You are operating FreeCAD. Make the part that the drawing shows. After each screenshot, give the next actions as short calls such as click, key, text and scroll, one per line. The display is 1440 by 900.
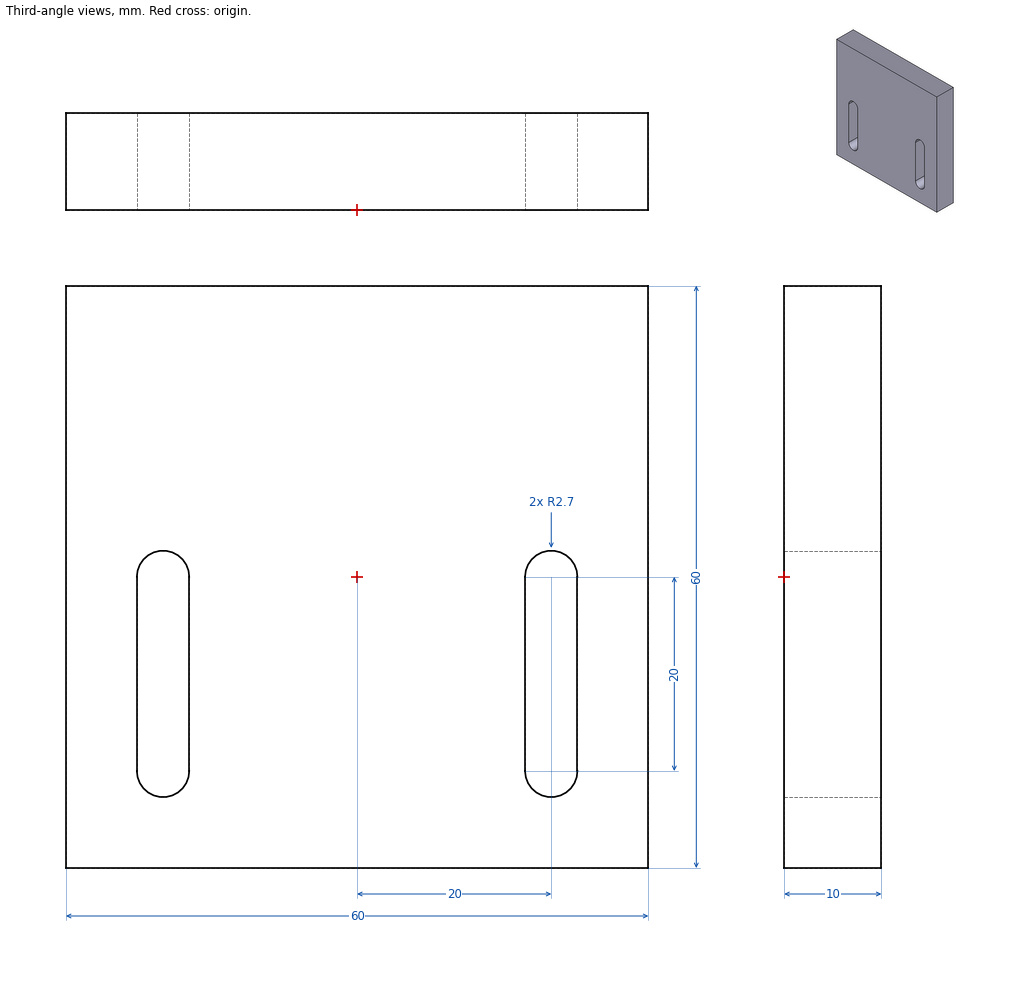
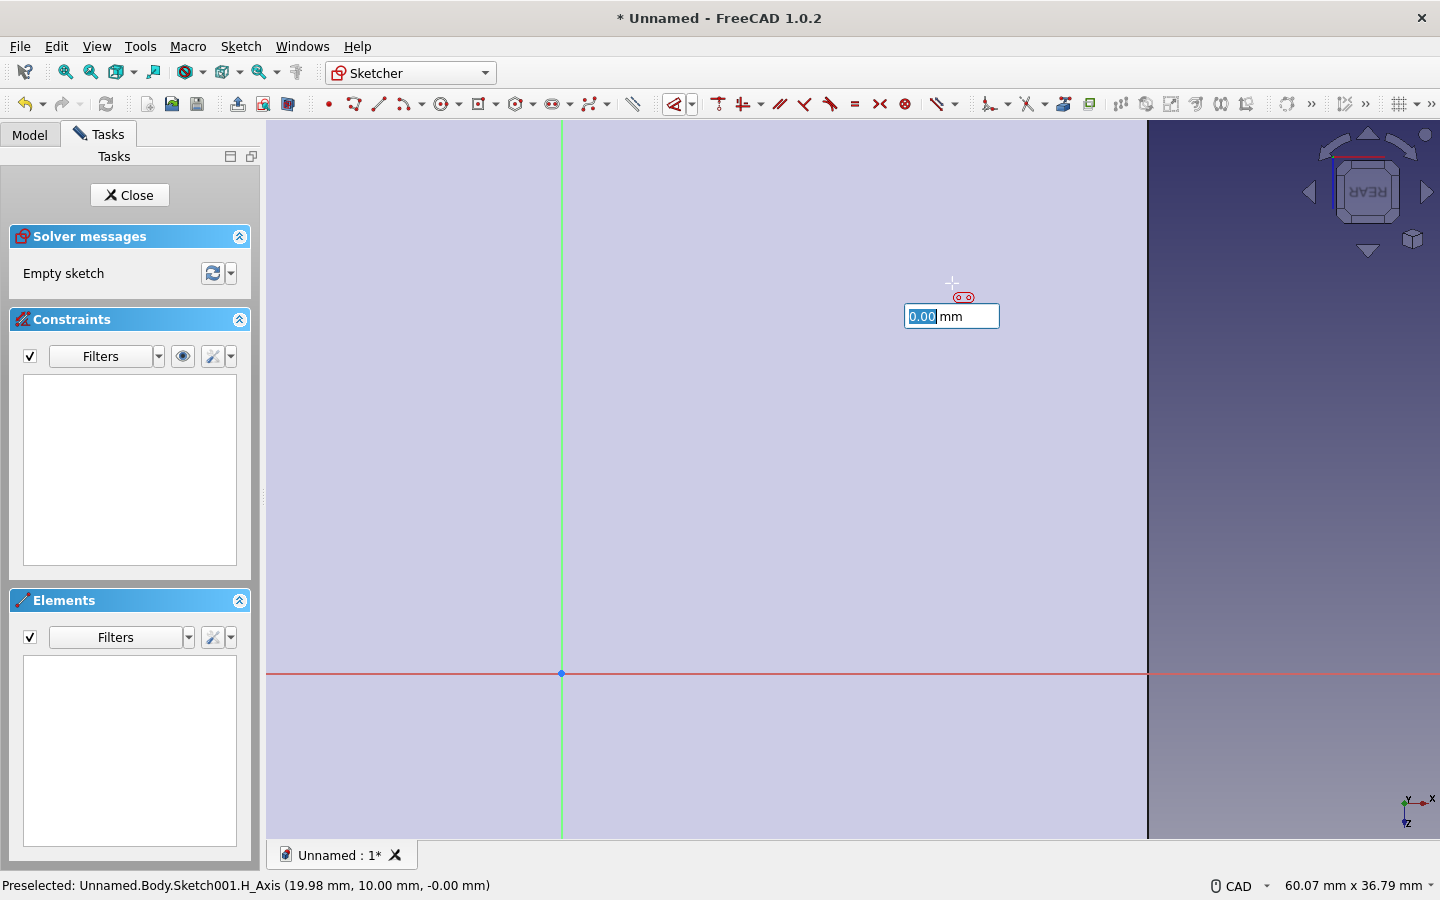
click(900, 478)
key(Escape)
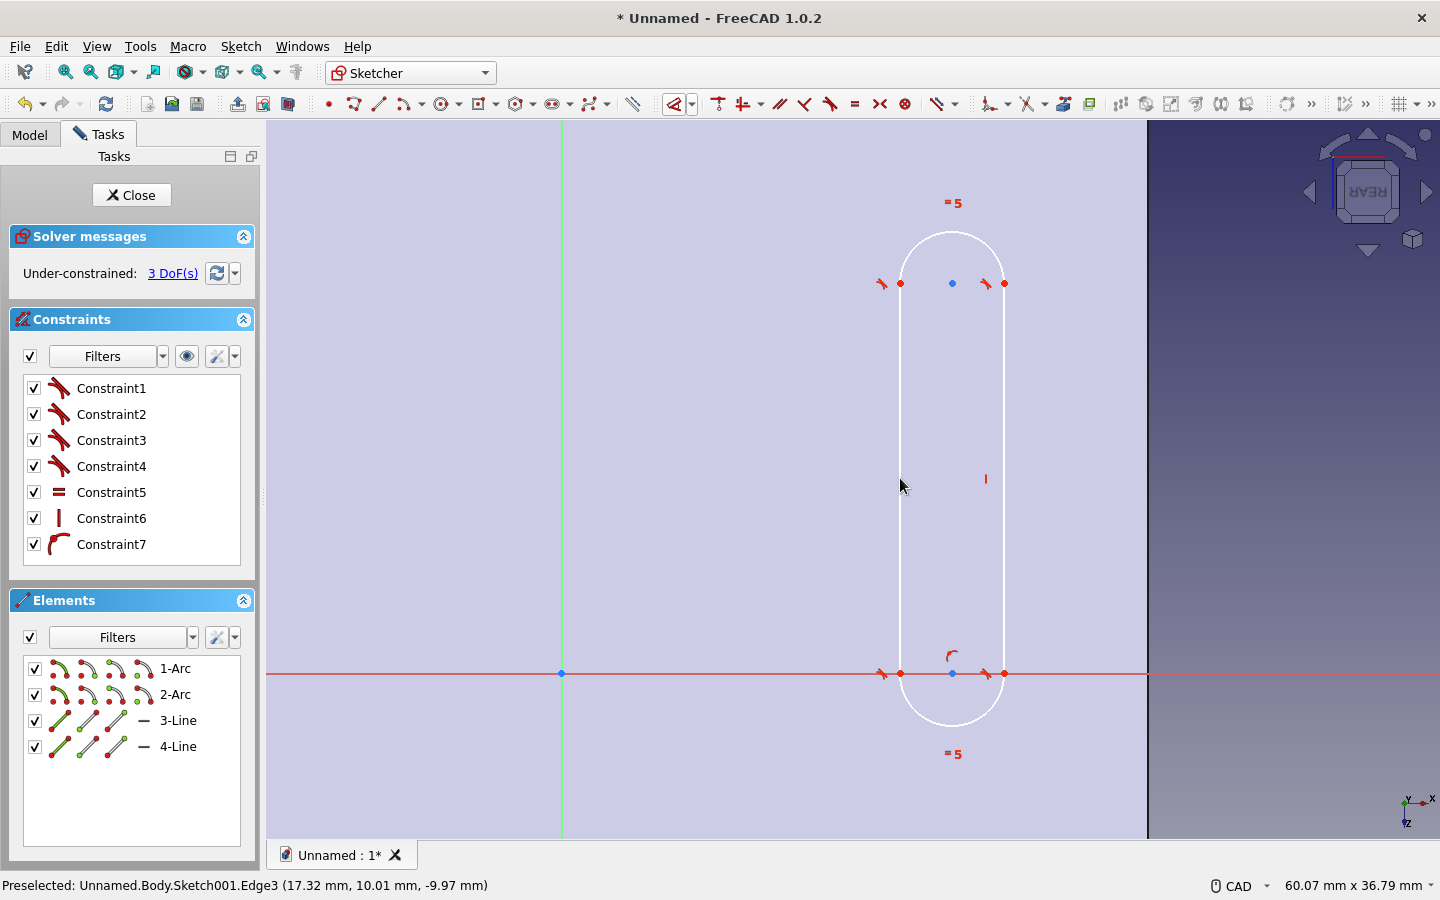
click(921, 716)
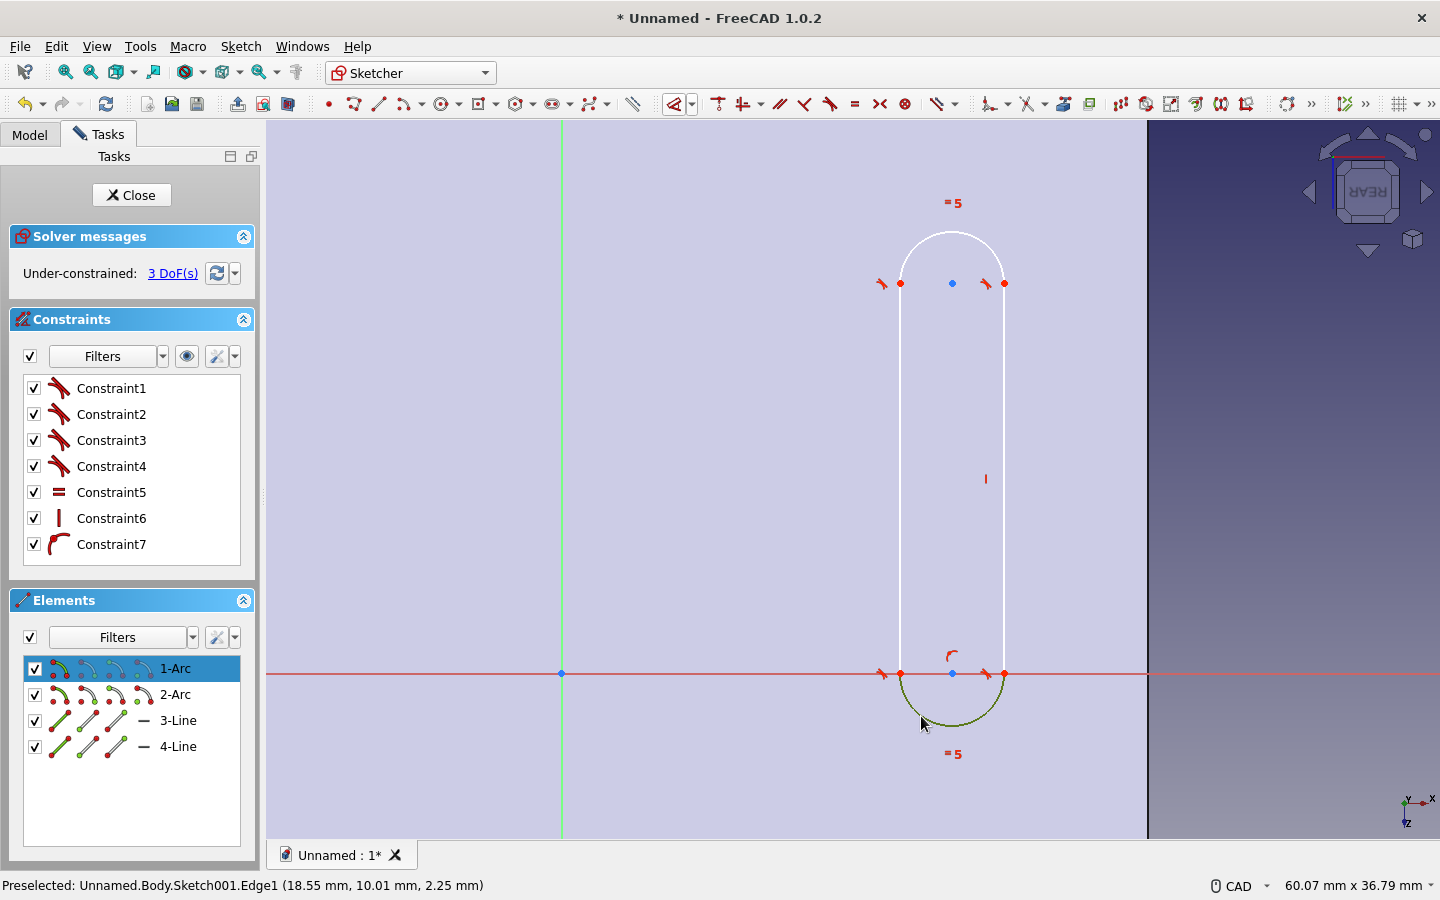
key(k)
key(r)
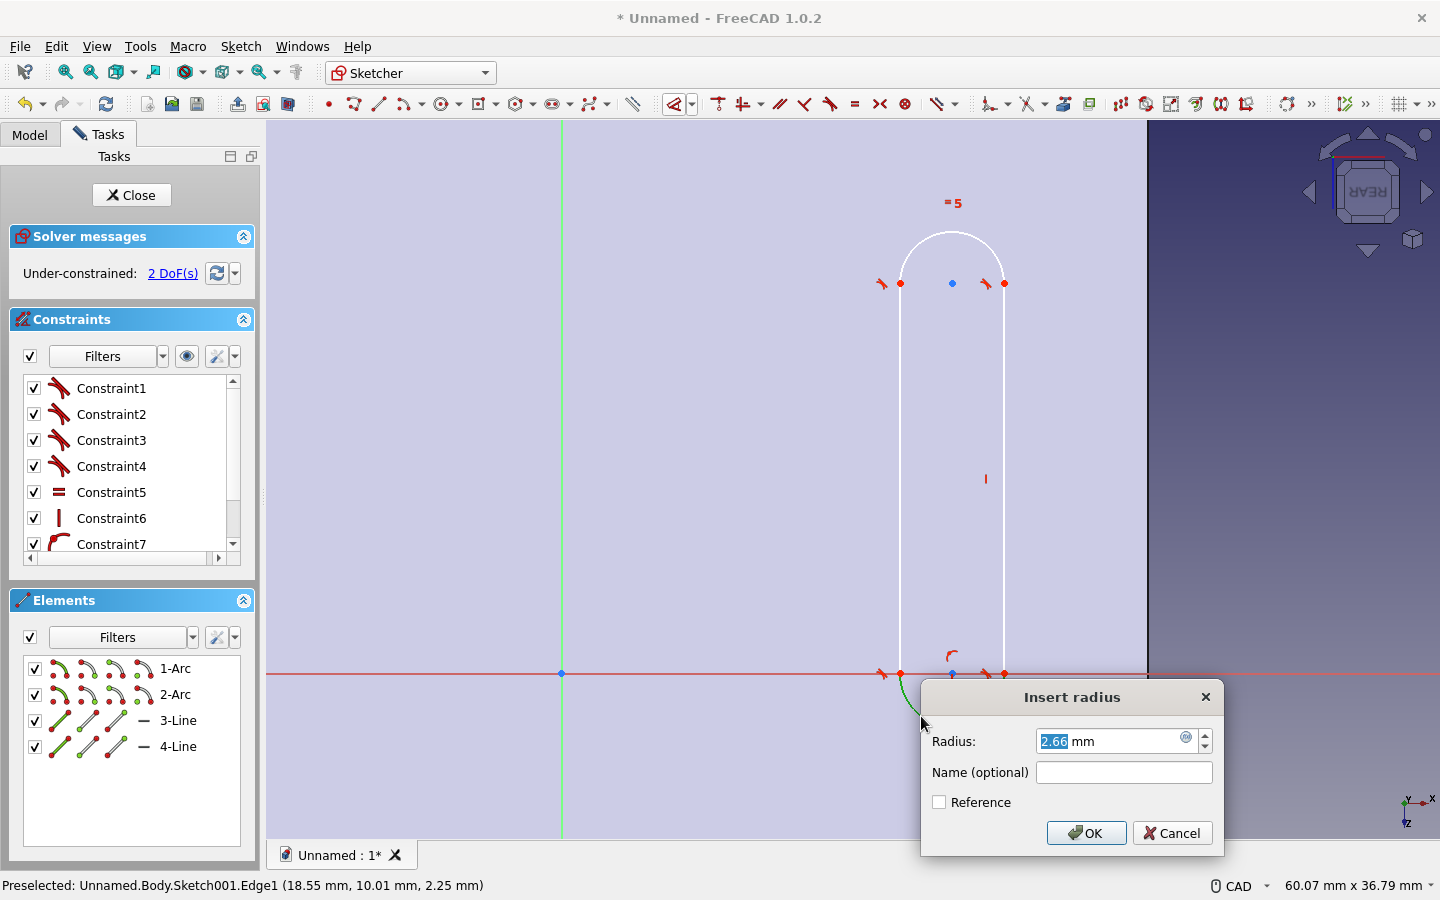
text(2.7)
key(Return)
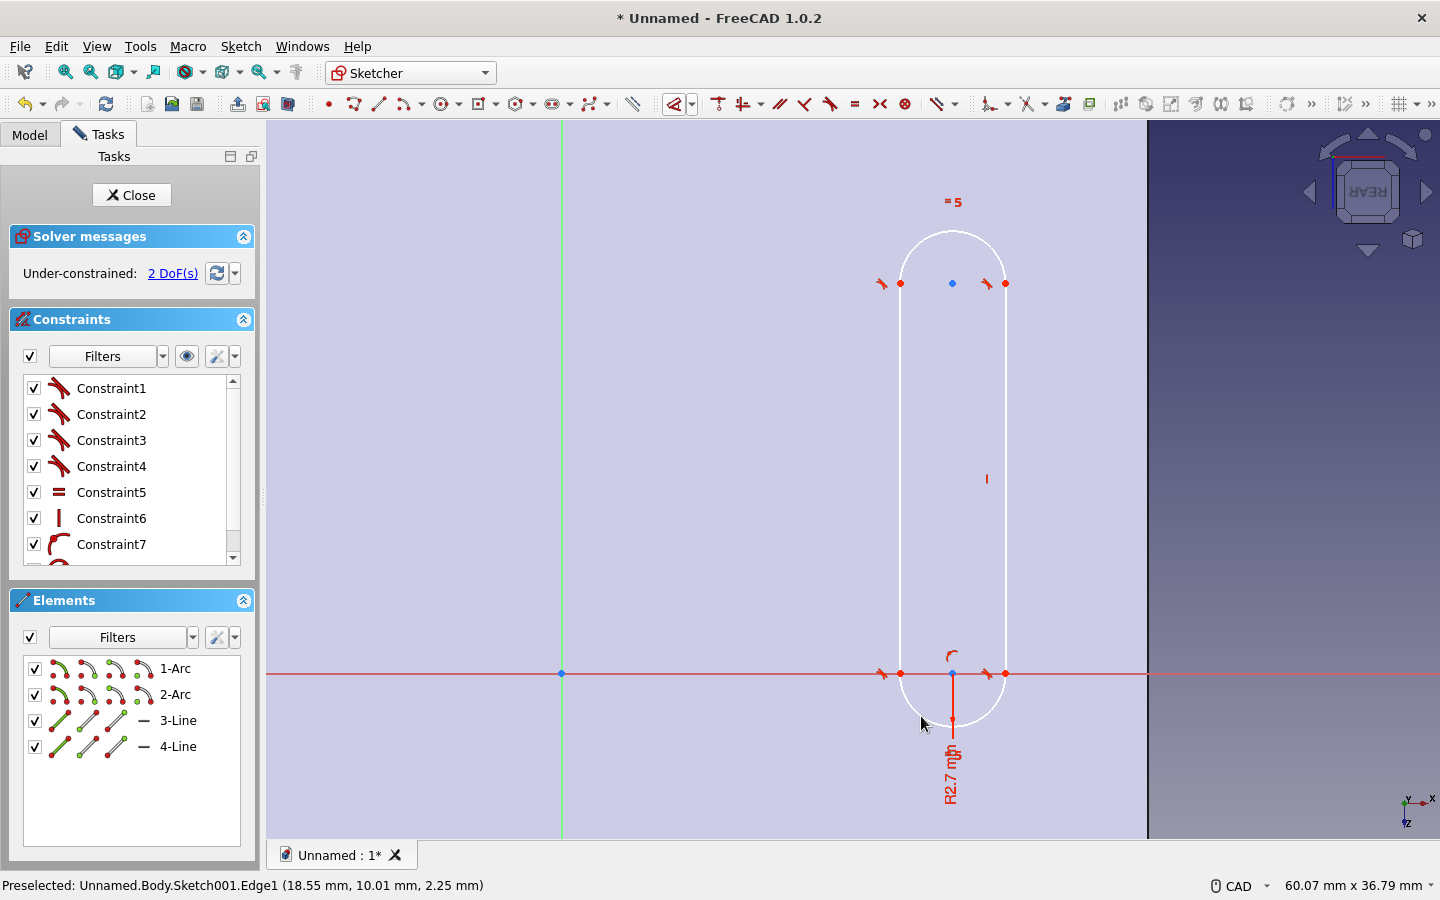
click(900, 557)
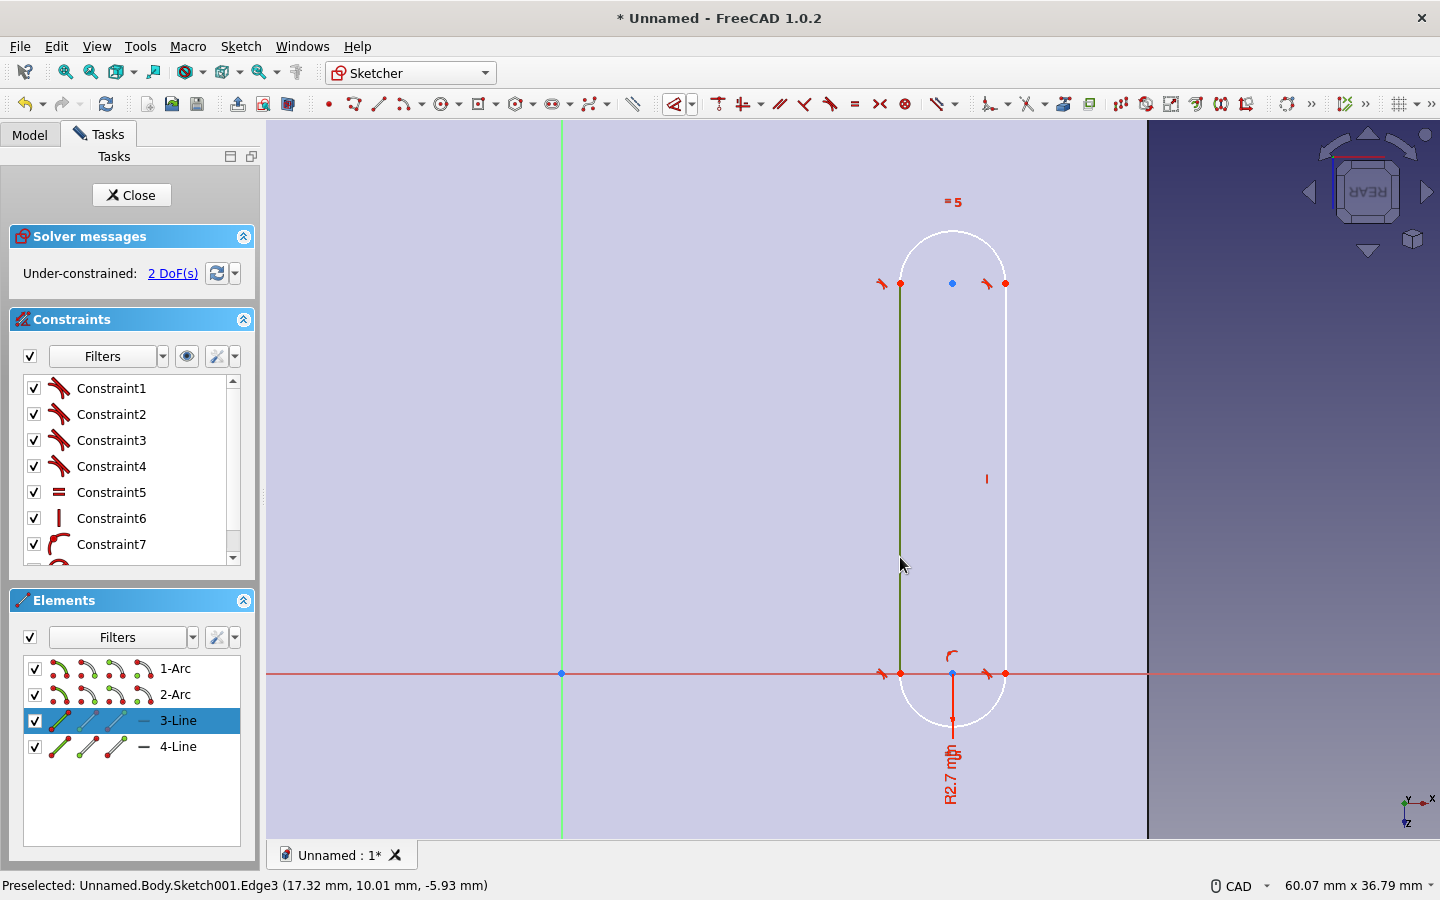
key(i)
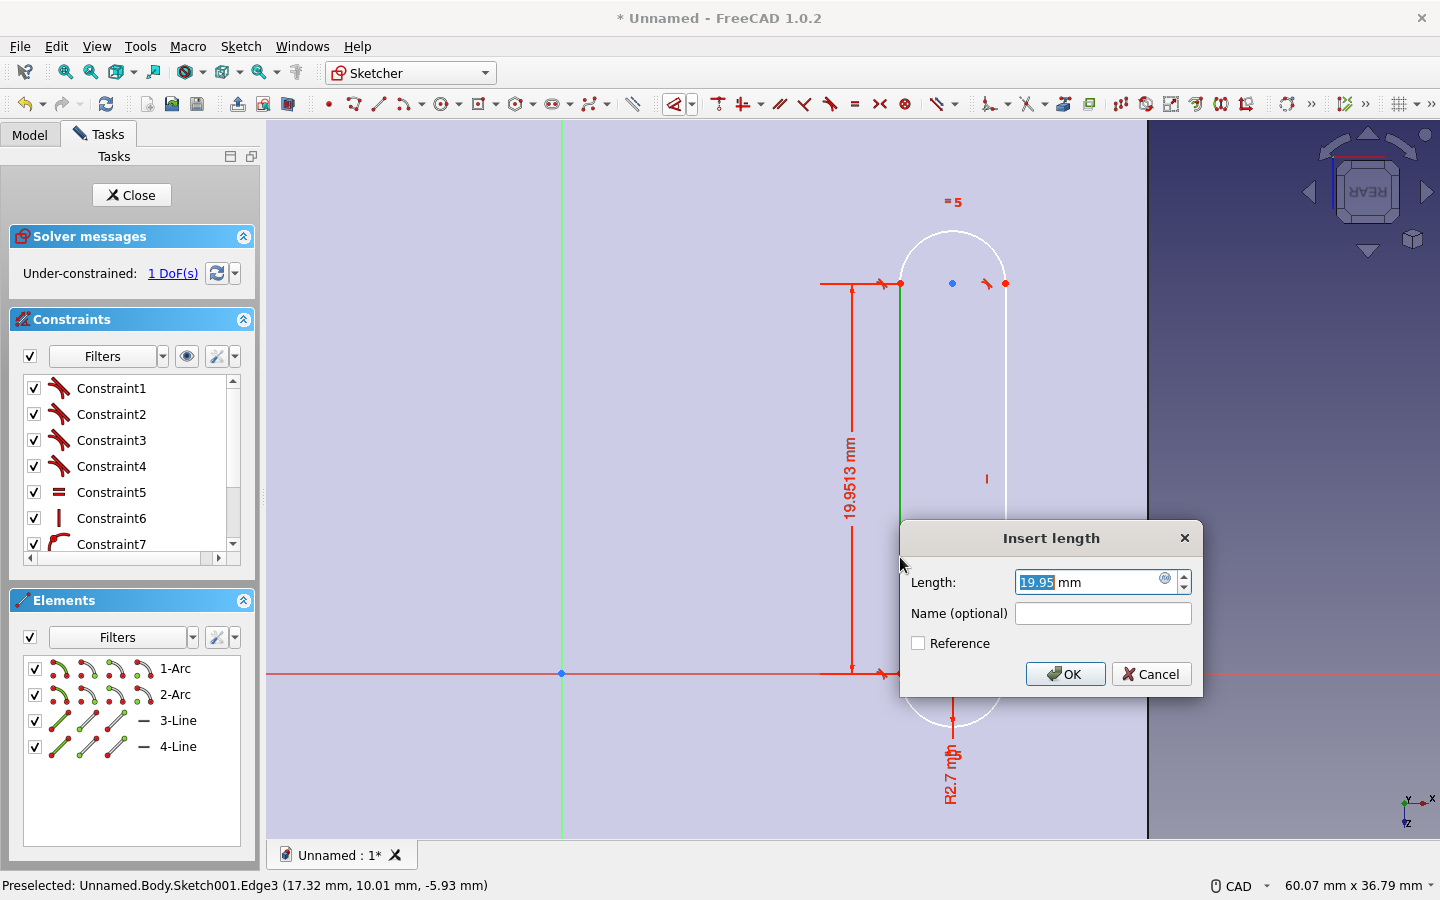
text(20)
key(Return)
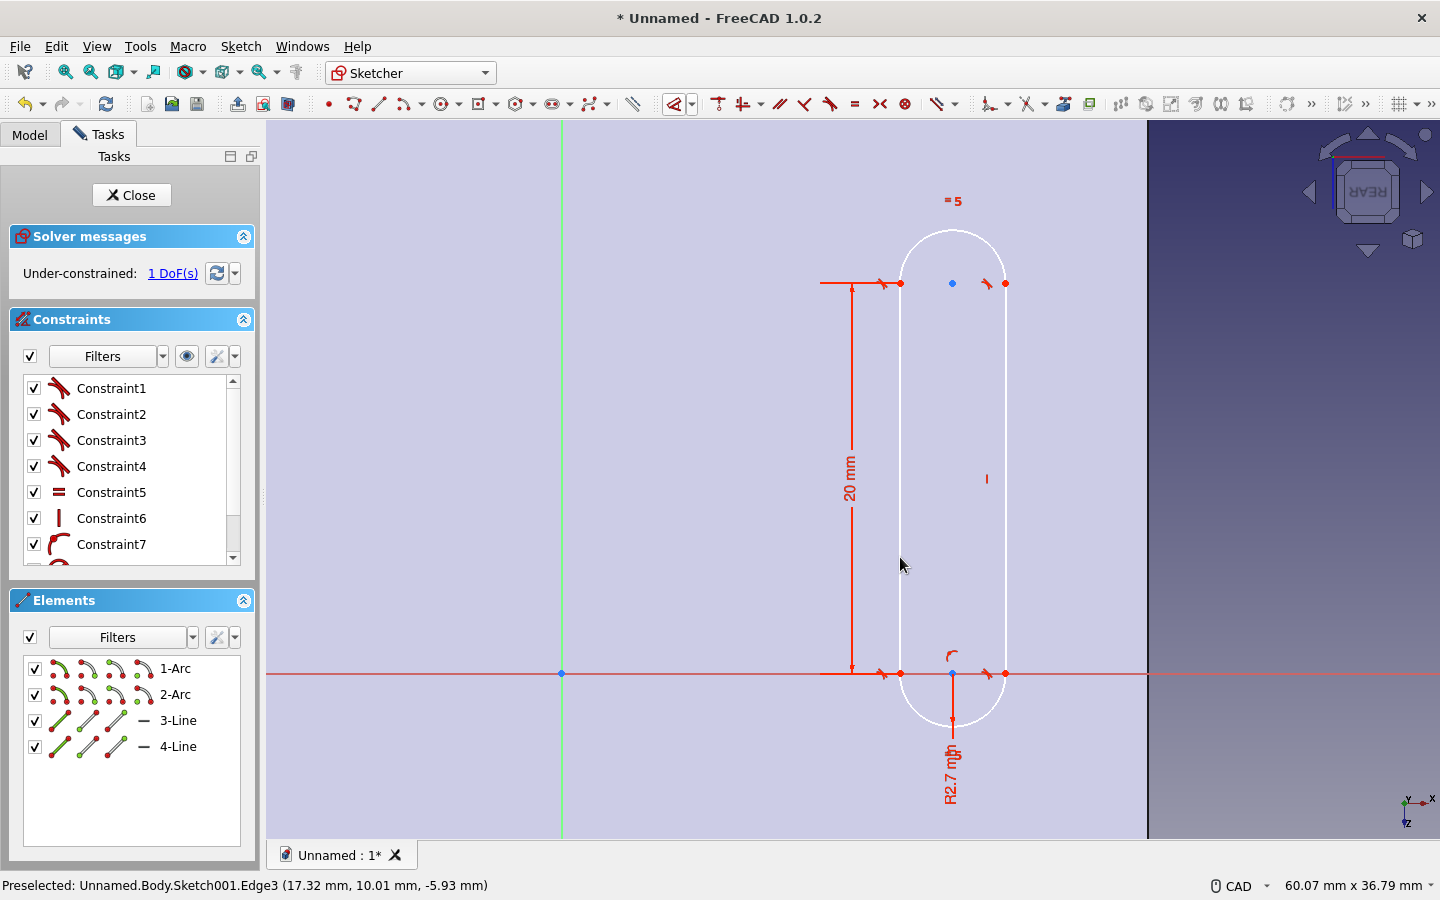
click(953, 674)